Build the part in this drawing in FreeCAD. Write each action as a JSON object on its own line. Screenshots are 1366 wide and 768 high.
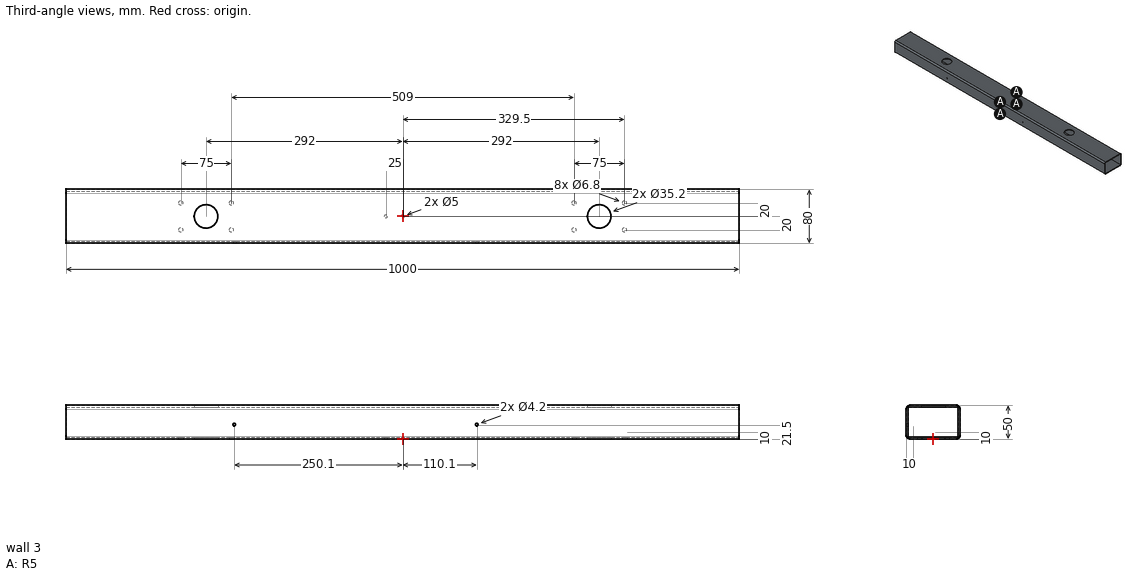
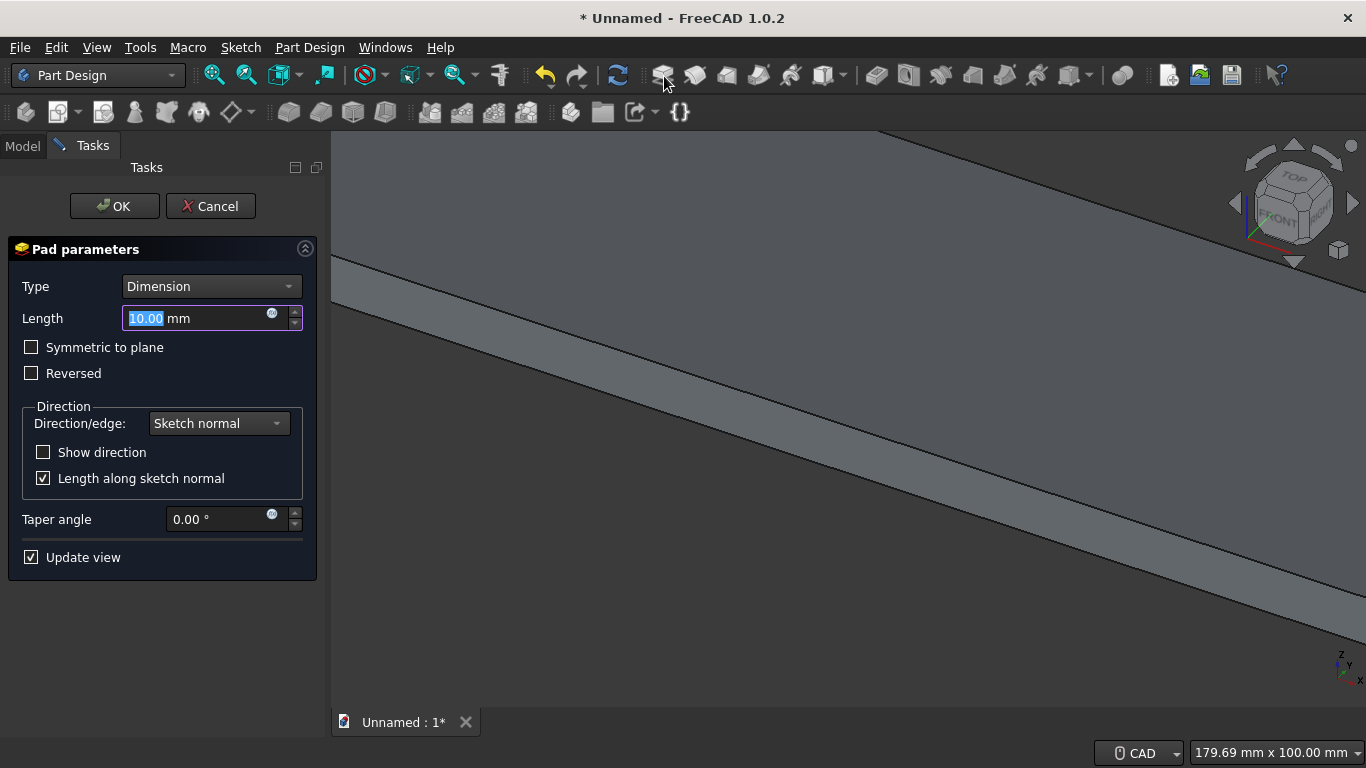
{"action": "type", "text": "50"}
{"action": "key", "text": "Tab"}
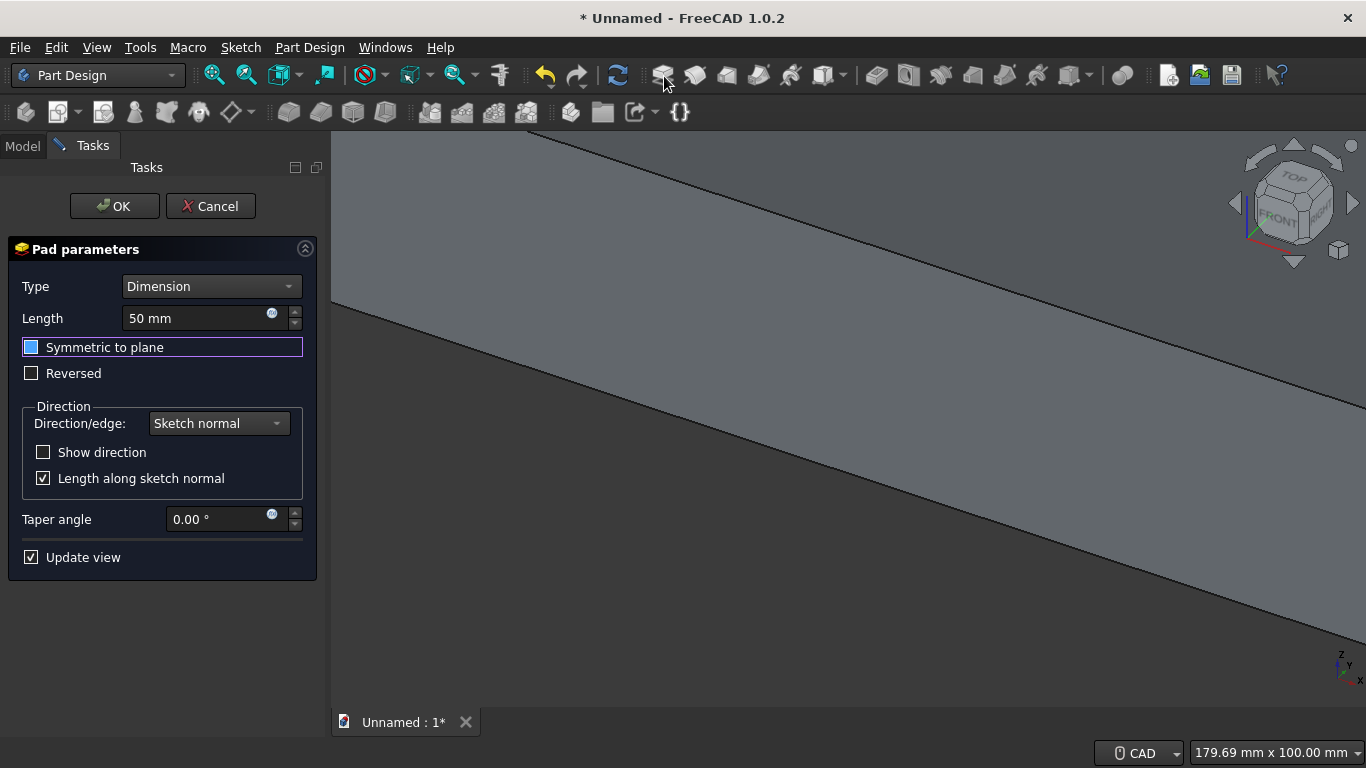
{"action": "left_click", "coordinate": [115, 206]}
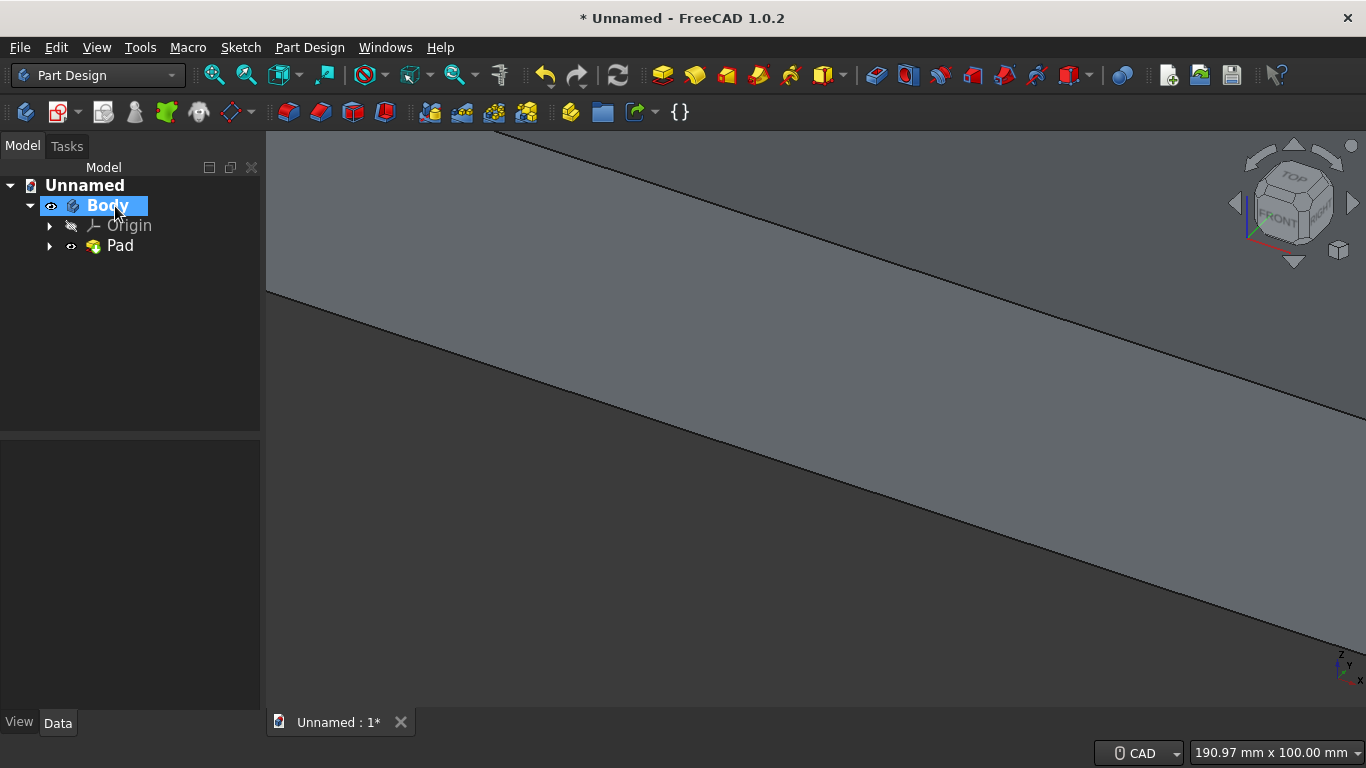
{"action": "left_click", "coordinate": [216, 76]}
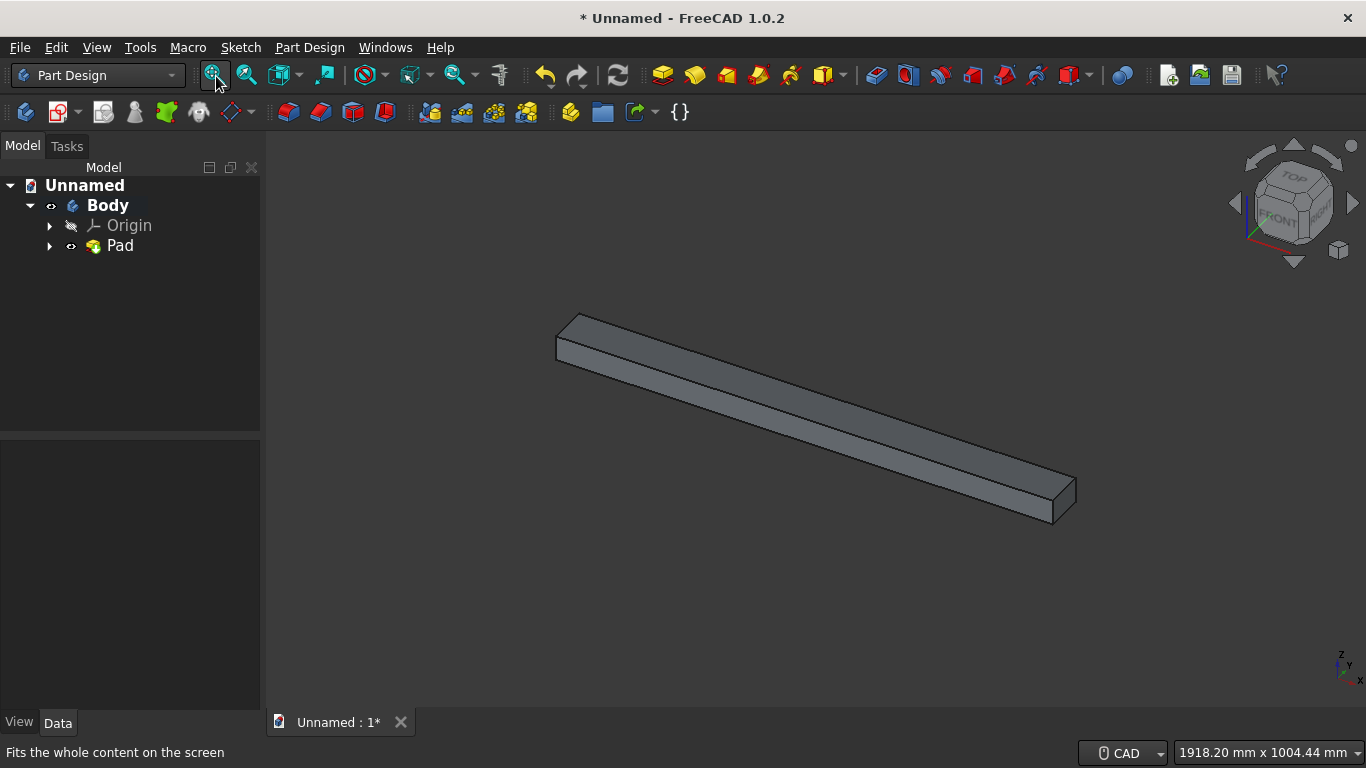
{"action": "left_click", "coordinate": [1068, 500]}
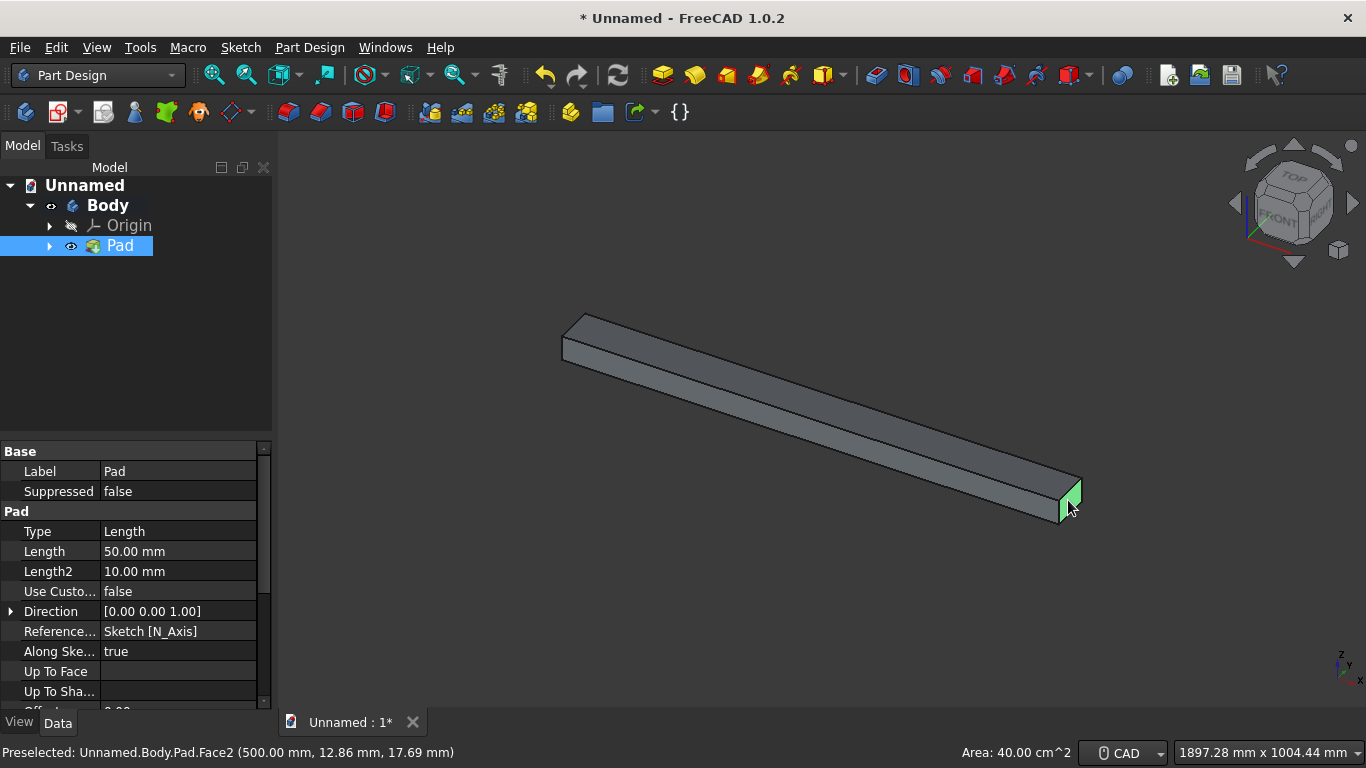
{"action": "key", "text": "0"}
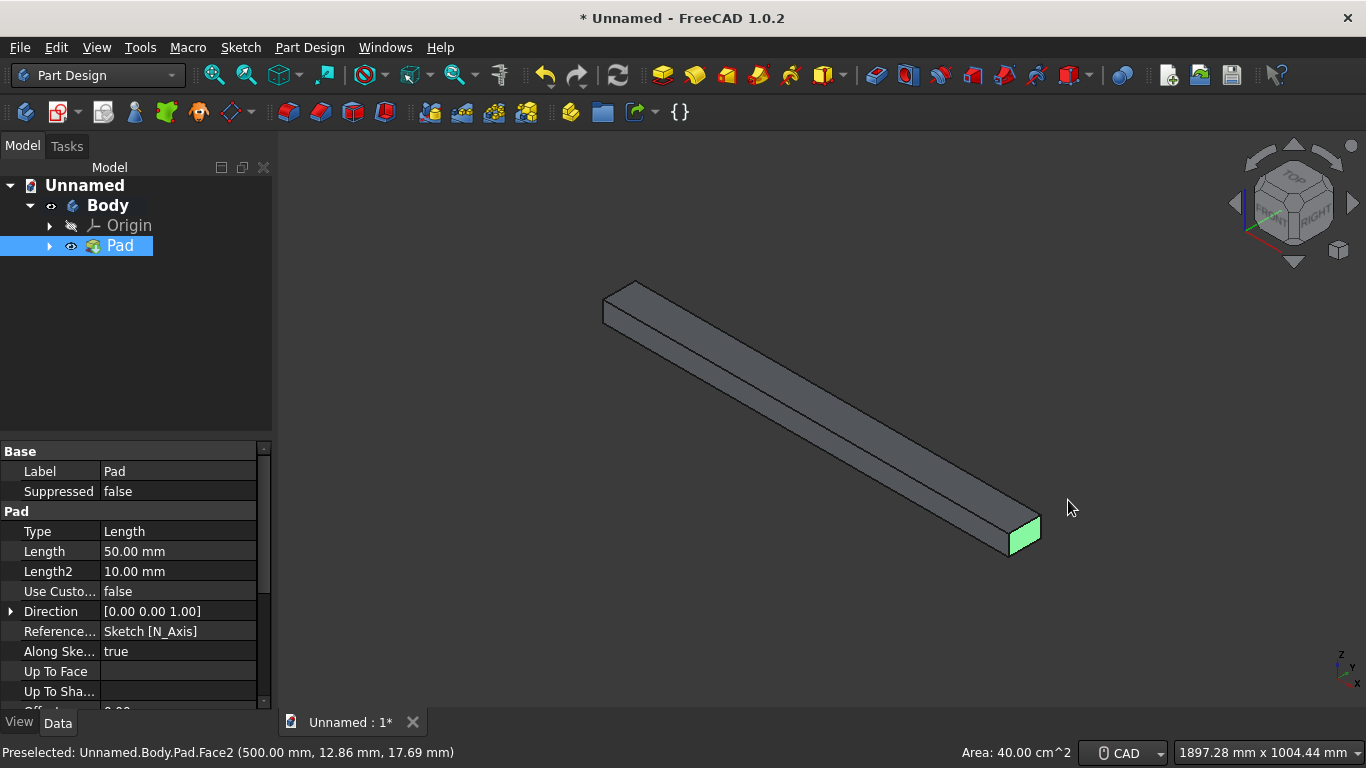
{"action": "key", "text": "2"}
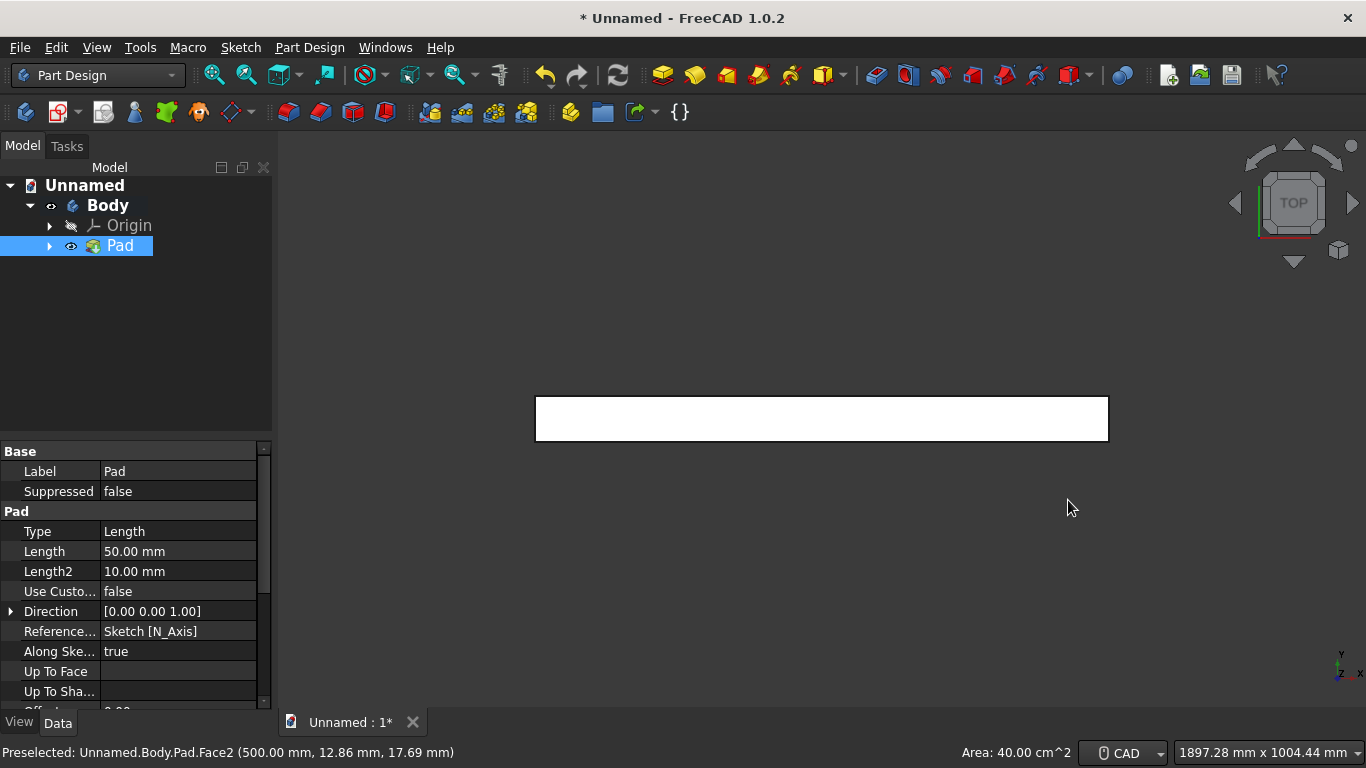
{"action": "key", "text": "1"}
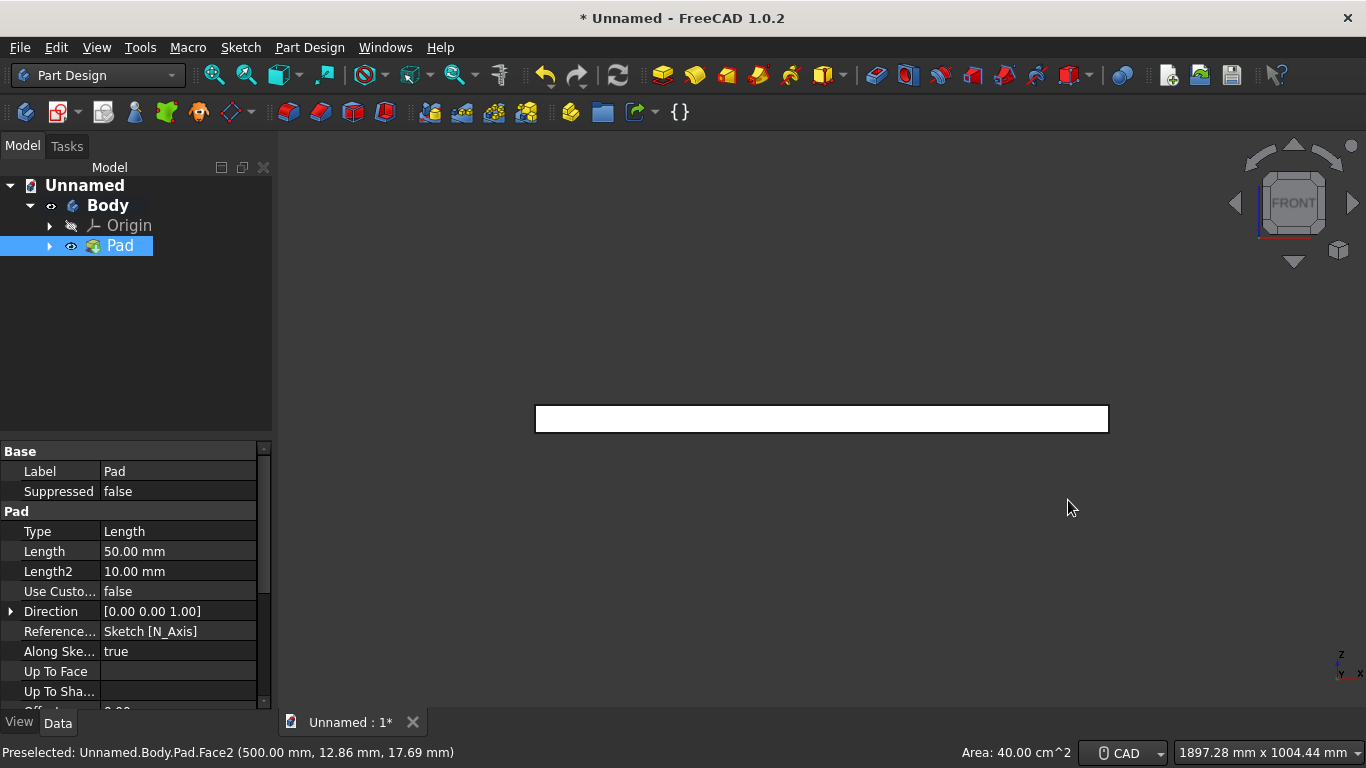
{"action": "key", "text": "3"}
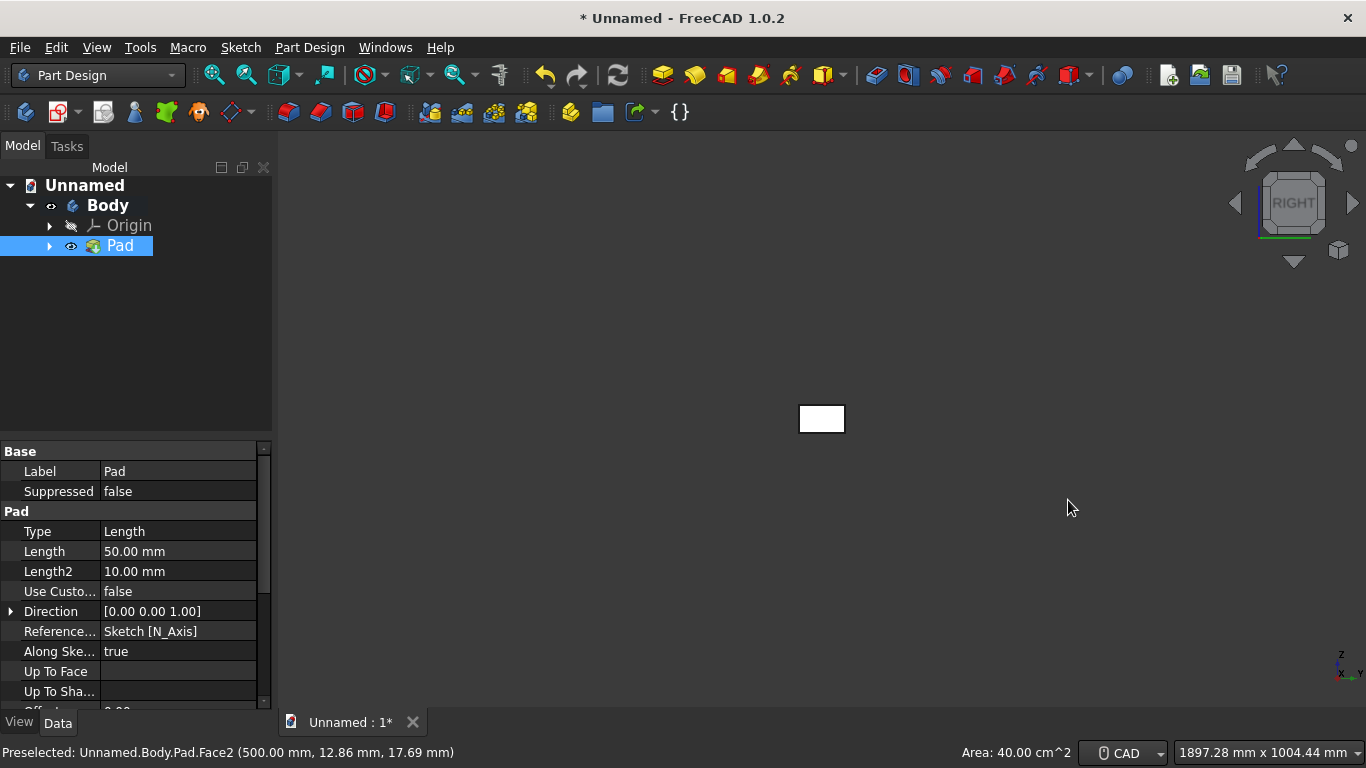
{"action": "left_click", "coordinate": [216, 76]}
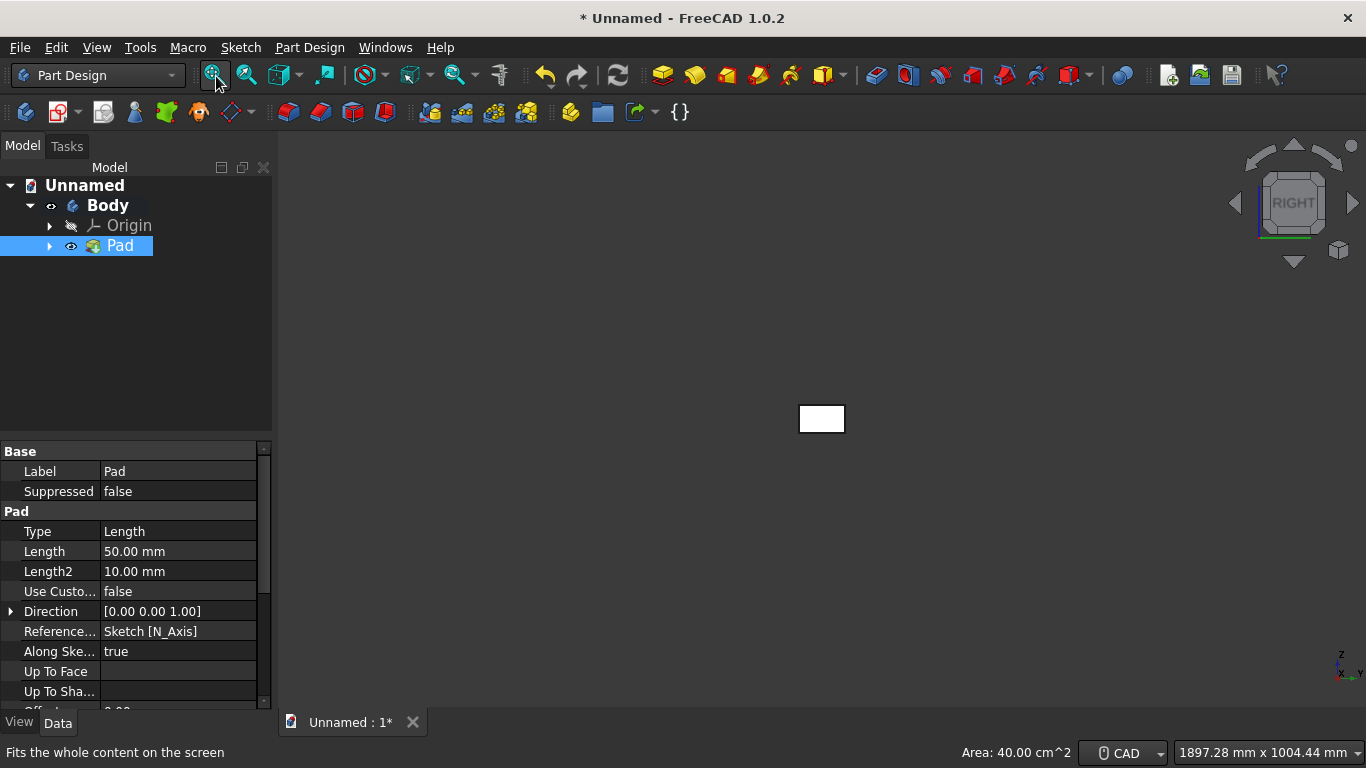
{"action": "key", "text": "5"}